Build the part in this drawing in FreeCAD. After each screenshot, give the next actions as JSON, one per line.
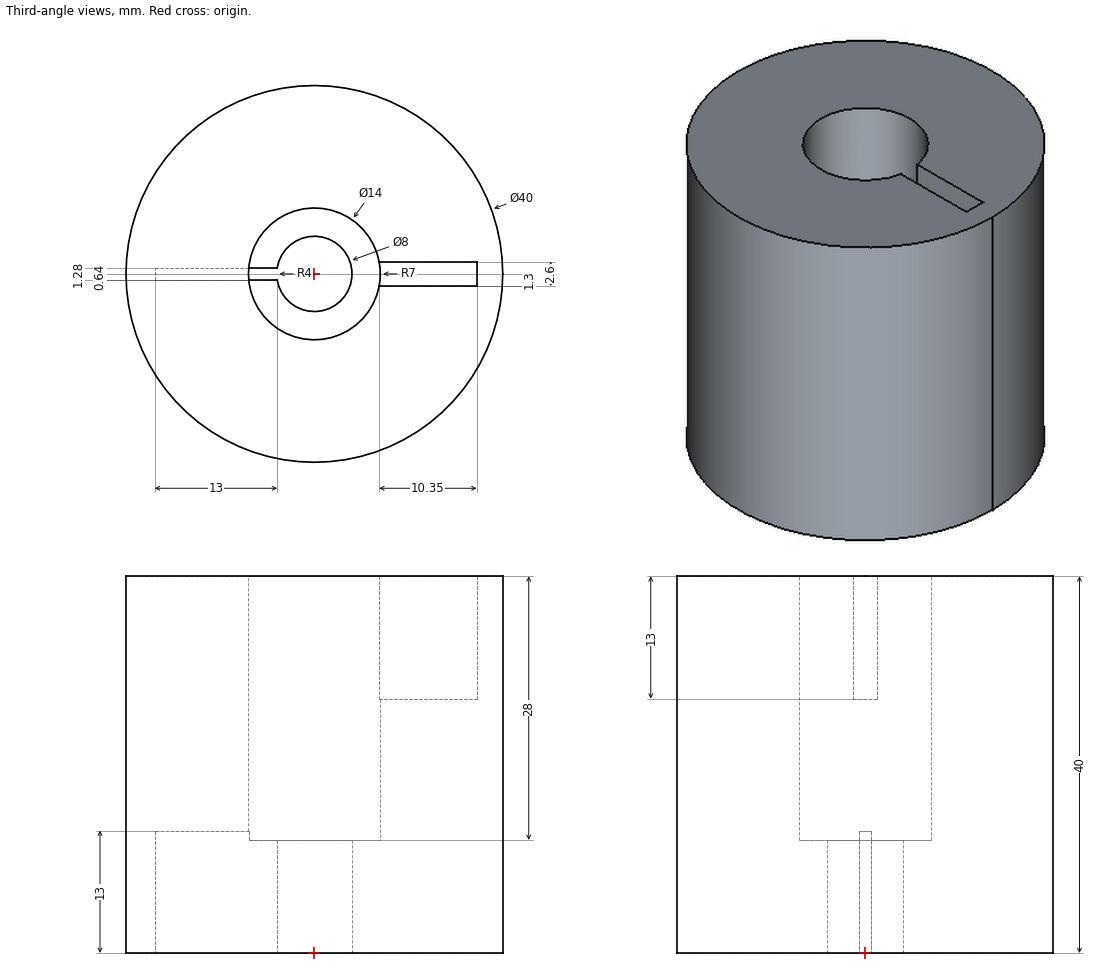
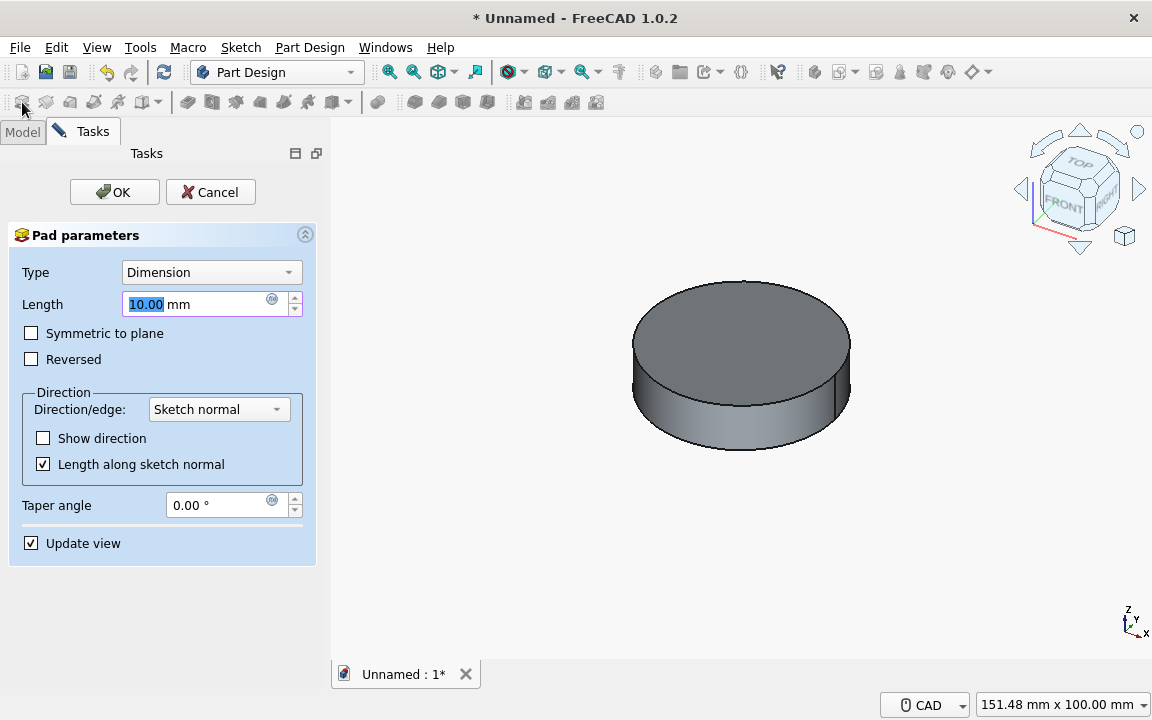
{"action": "type", "text": "40"}
{"action": "key", "text": "Tab"}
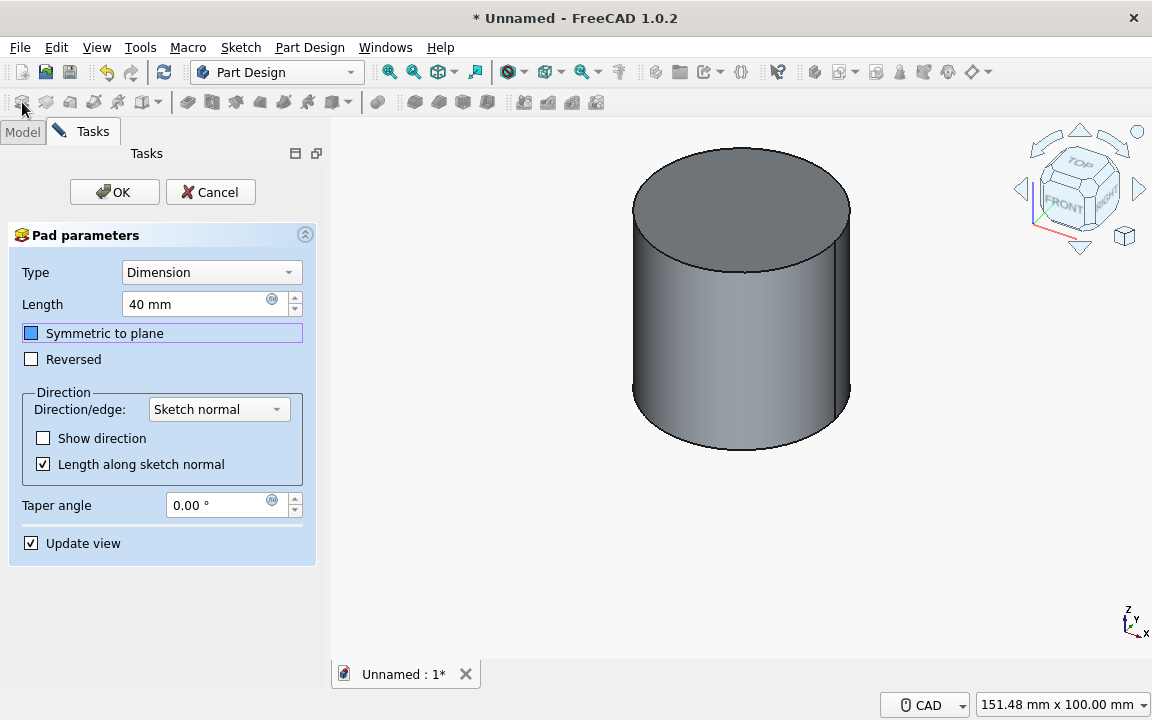
{"action": "left_click", "coordinate": [115, 192]}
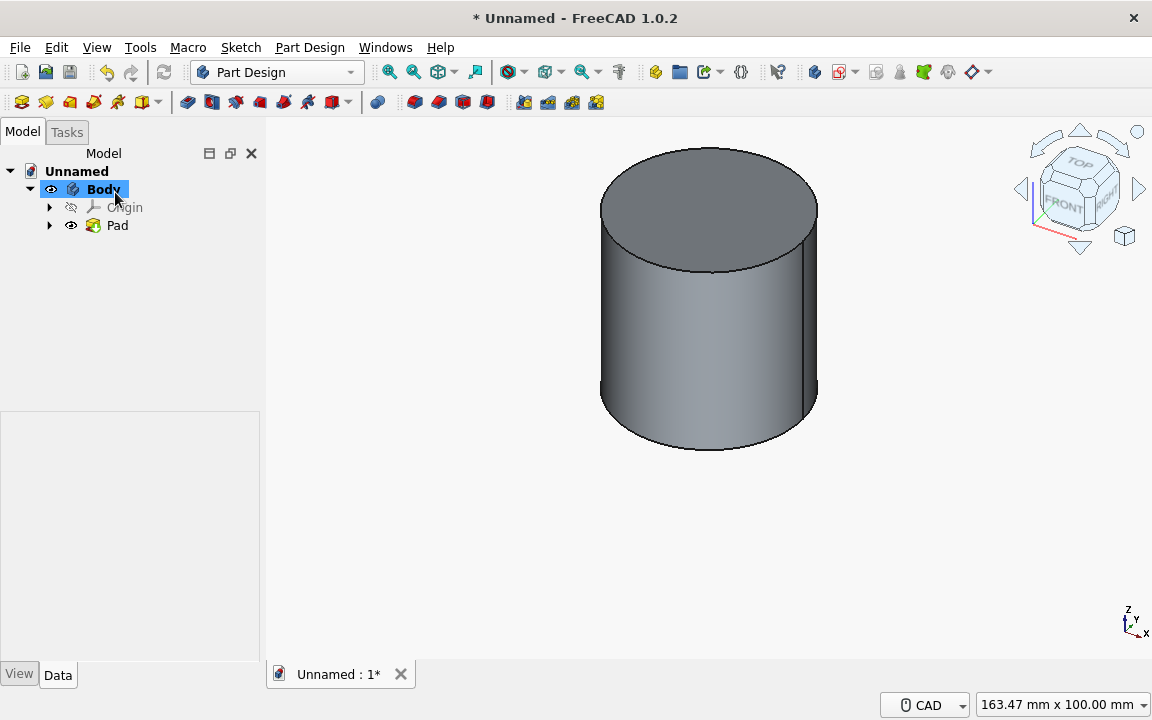
{"action": "left_click", "coordinate": [709, 209]}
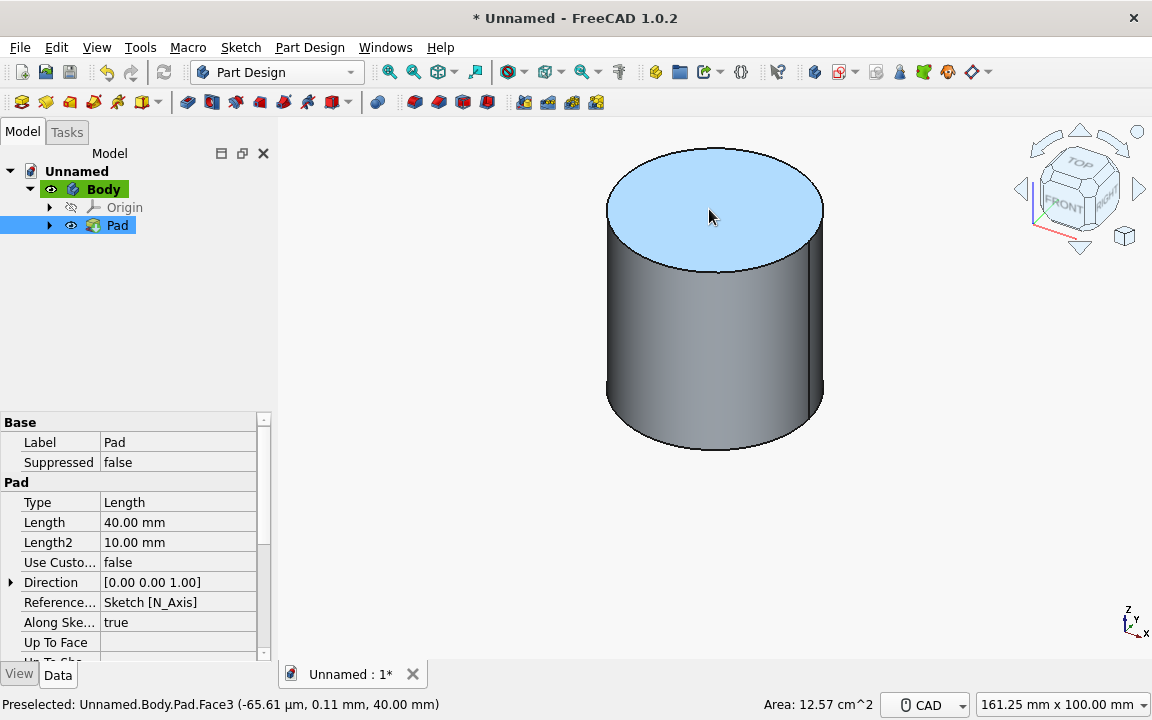
{"action": "left_click", "coordinate": [840, 72]}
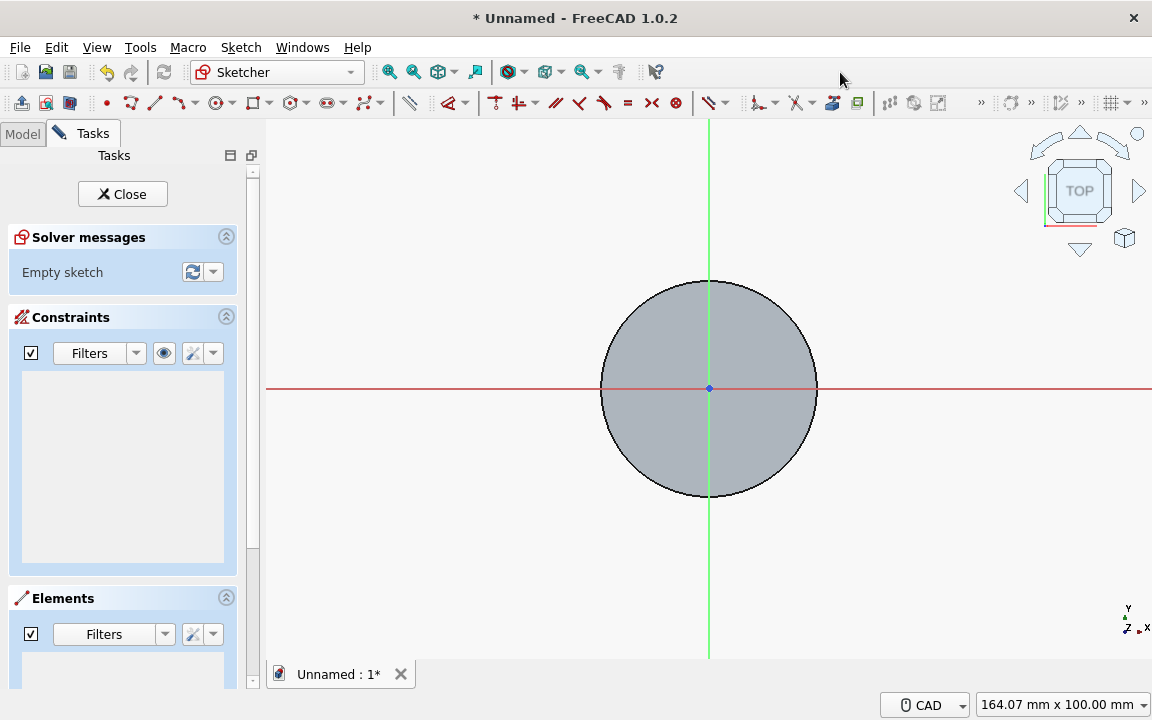
{"action": "scroll", "coordinate": [720, 389], "scroll_direction": "up", "scroll_amount": 10}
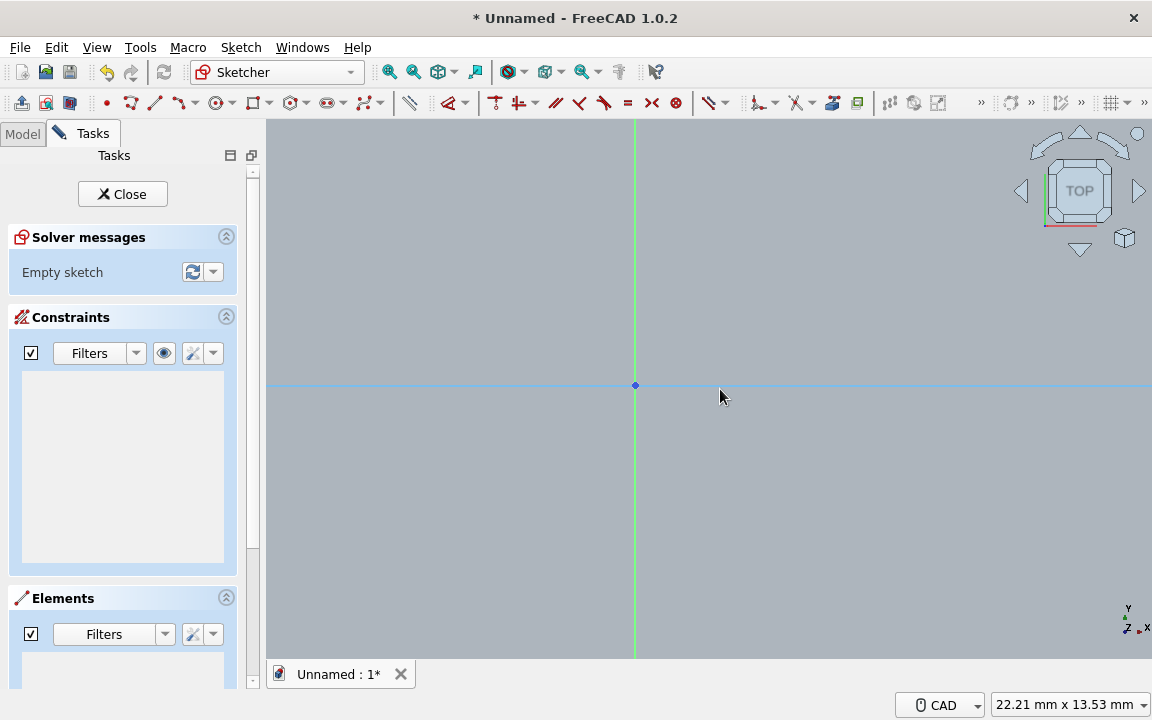
{"action": "key", "text": "g c"}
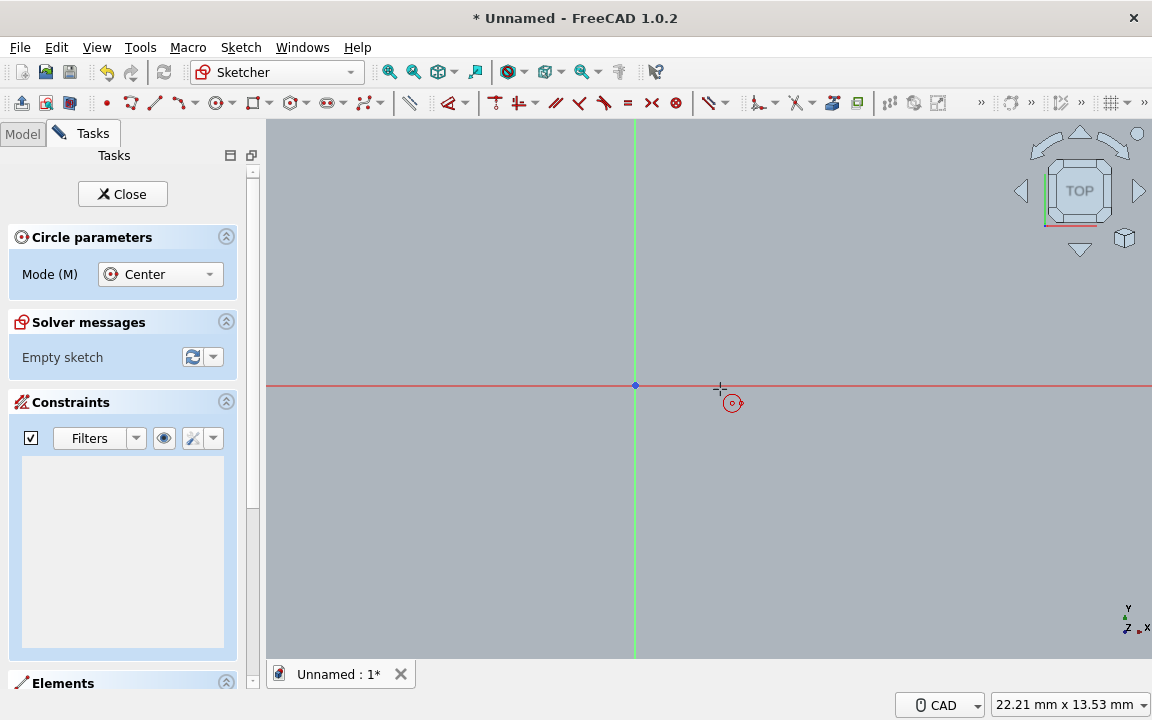
{"action": "left_click", "coordinate": [635, 386]}
{"action": "left_click", "coordinate": [748, 273]}
{"action": "key", "text": "Escape"}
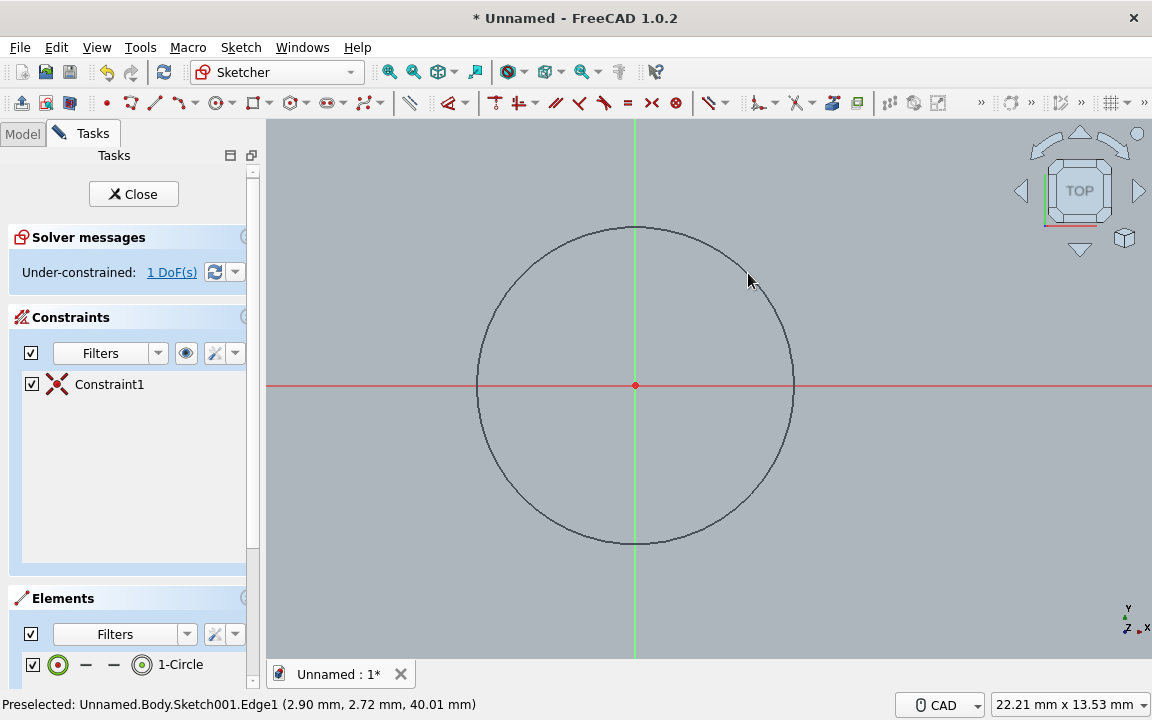
{"action": "left_click", "coordinate": [448, 104]}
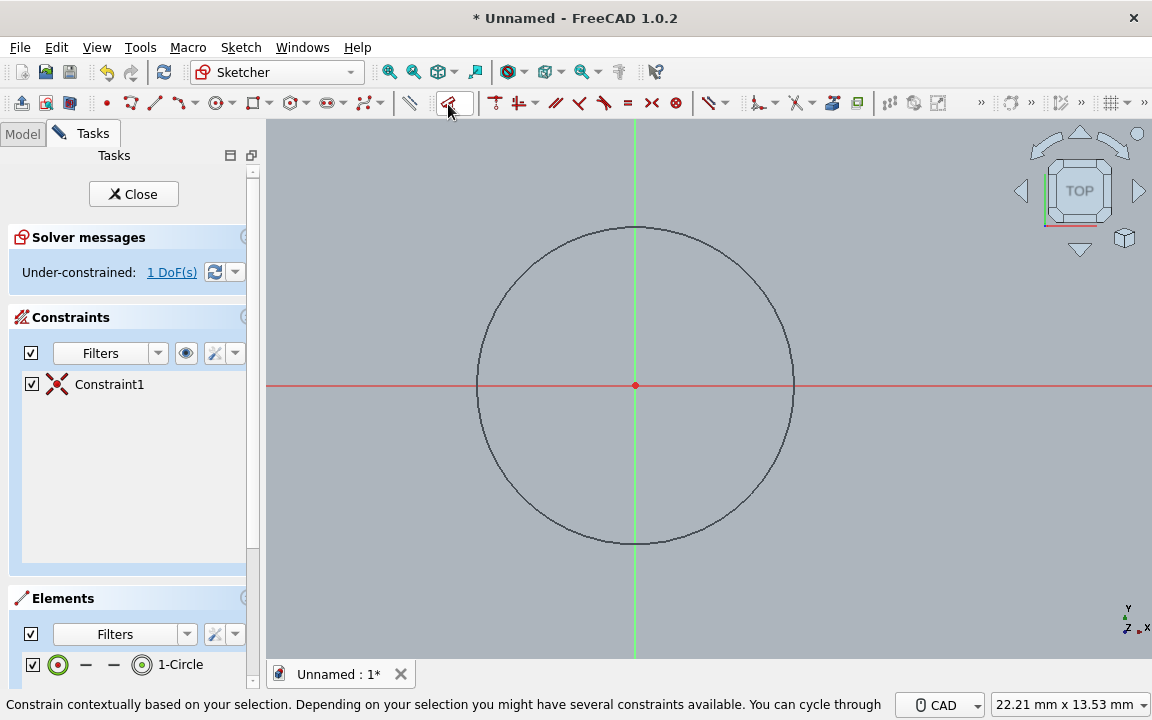
{"action": "left_click", "coordinate": [747, 273]}
{"action": "left_click", "coordinate": [770, 250]}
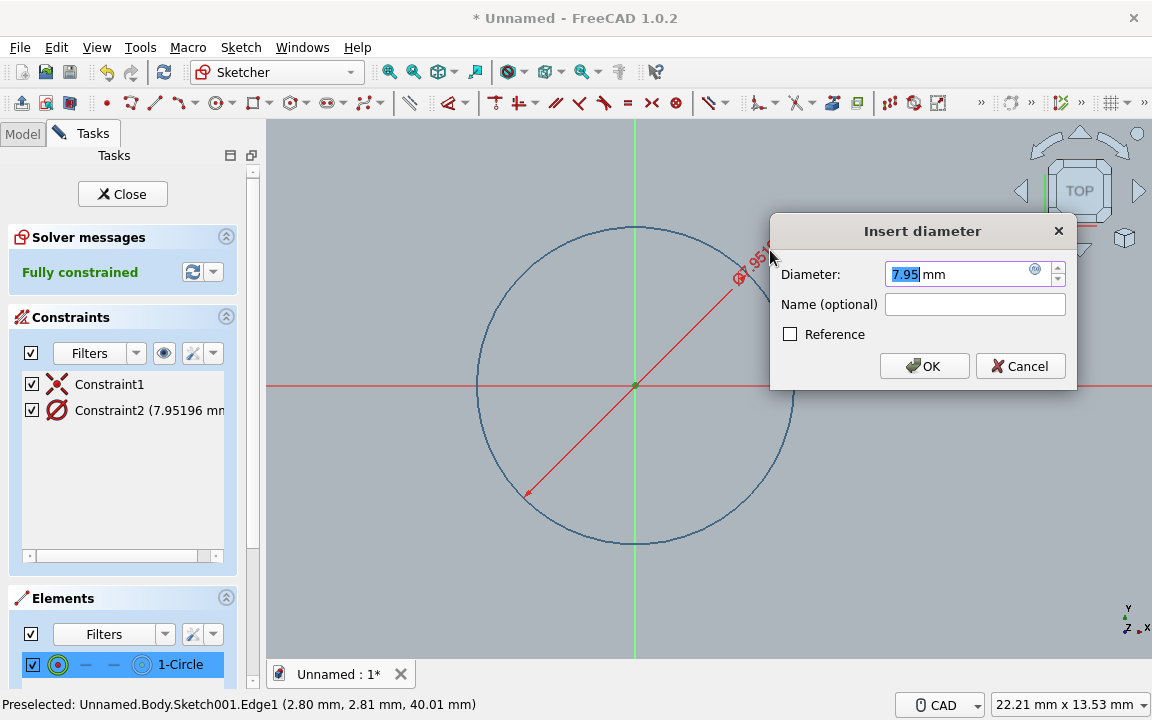
{"action": "type", "text": "8"}
{"action": "key", "text": "Return"}
{"action": "key", "text": "Escape"}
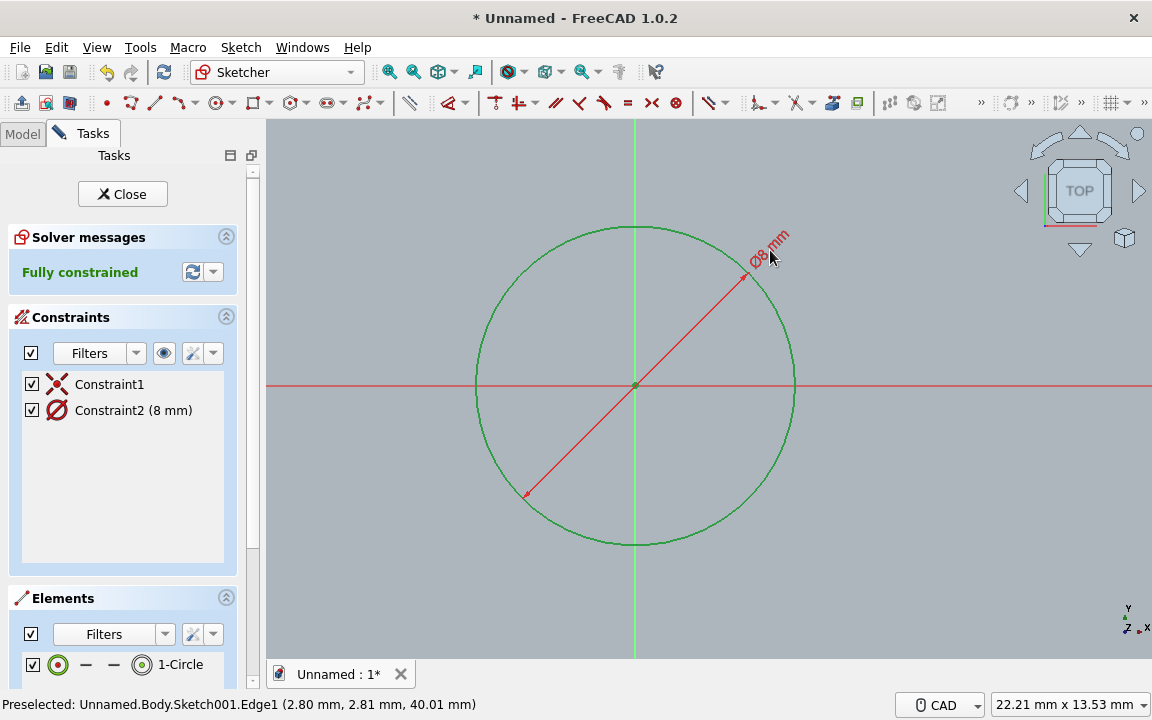
{"action": "left_click", "coordinate": [123, 194]}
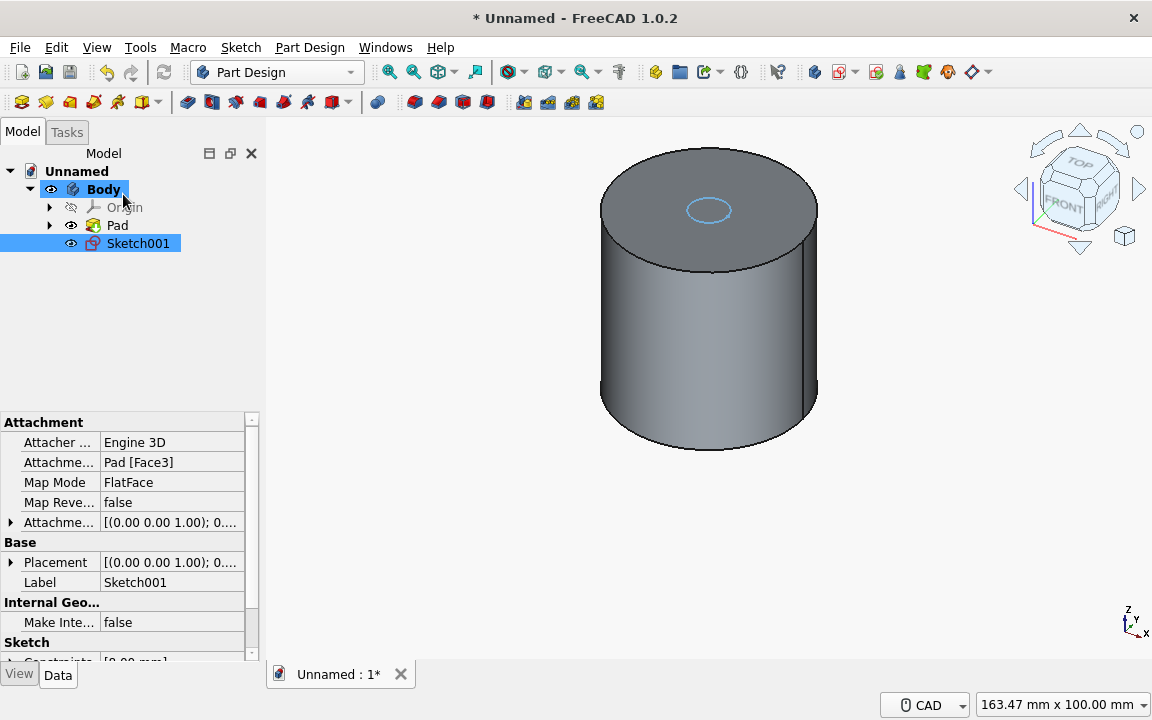
{"action": "left_click", "coordinate": [188, 102]}